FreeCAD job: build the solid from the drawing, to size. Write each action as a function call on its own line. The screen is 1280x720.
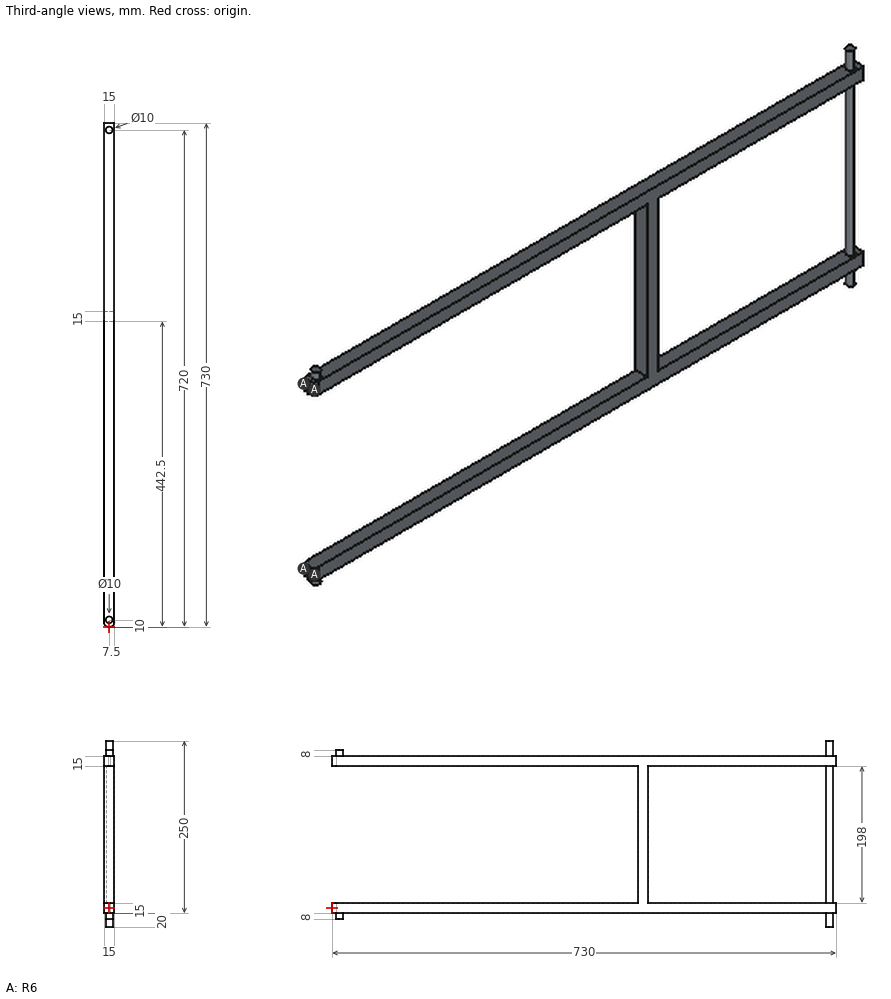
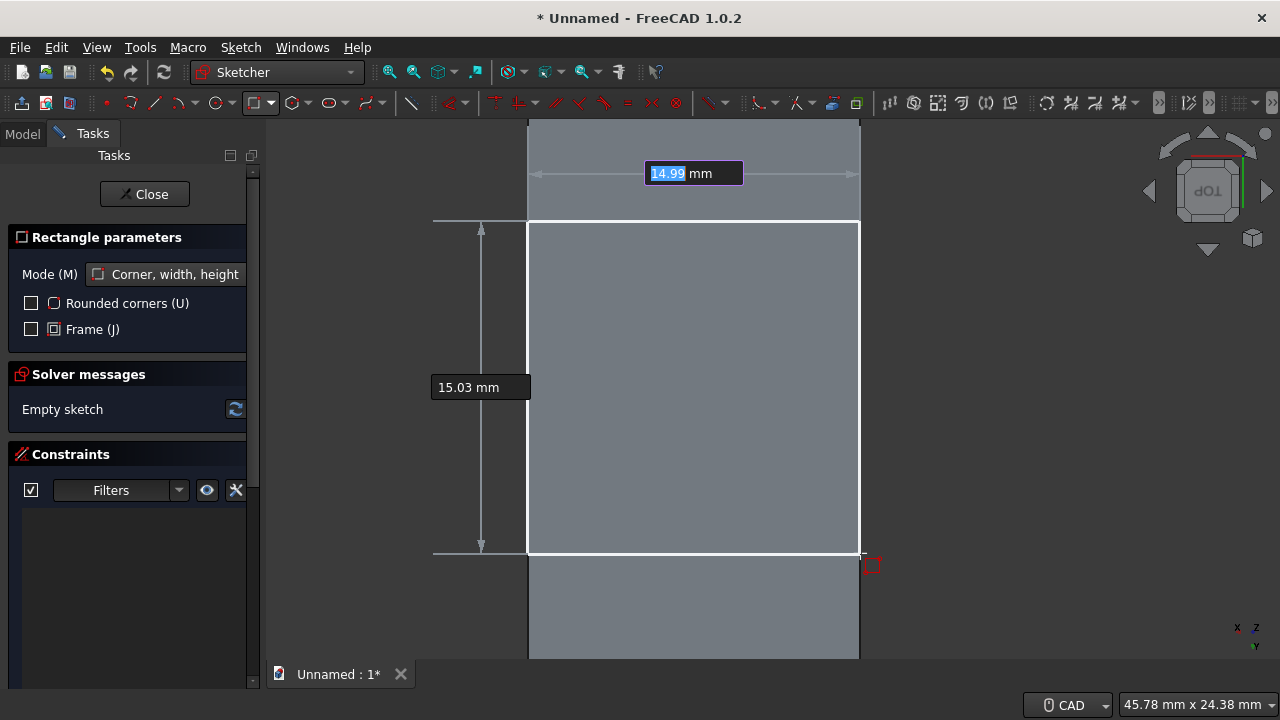
text(15)
key(Tab)
text(15)
key(Return)
key(Escape)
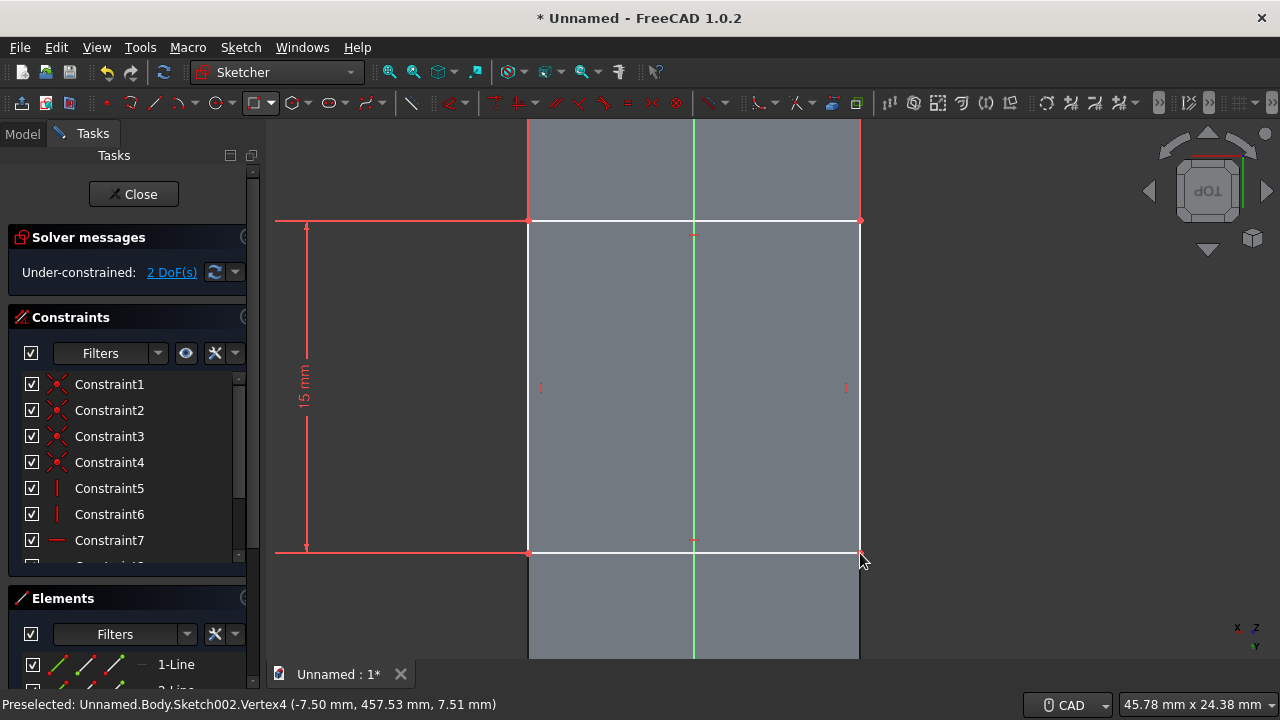
click(528, 221)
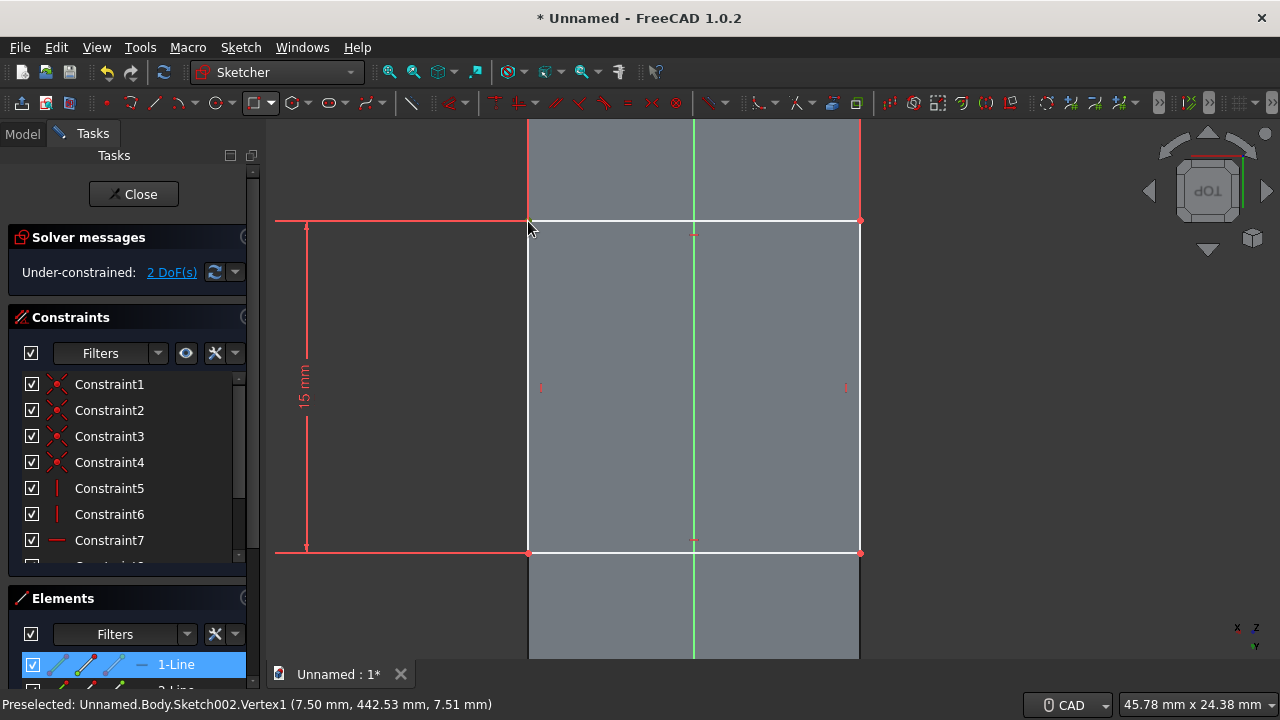
key(l)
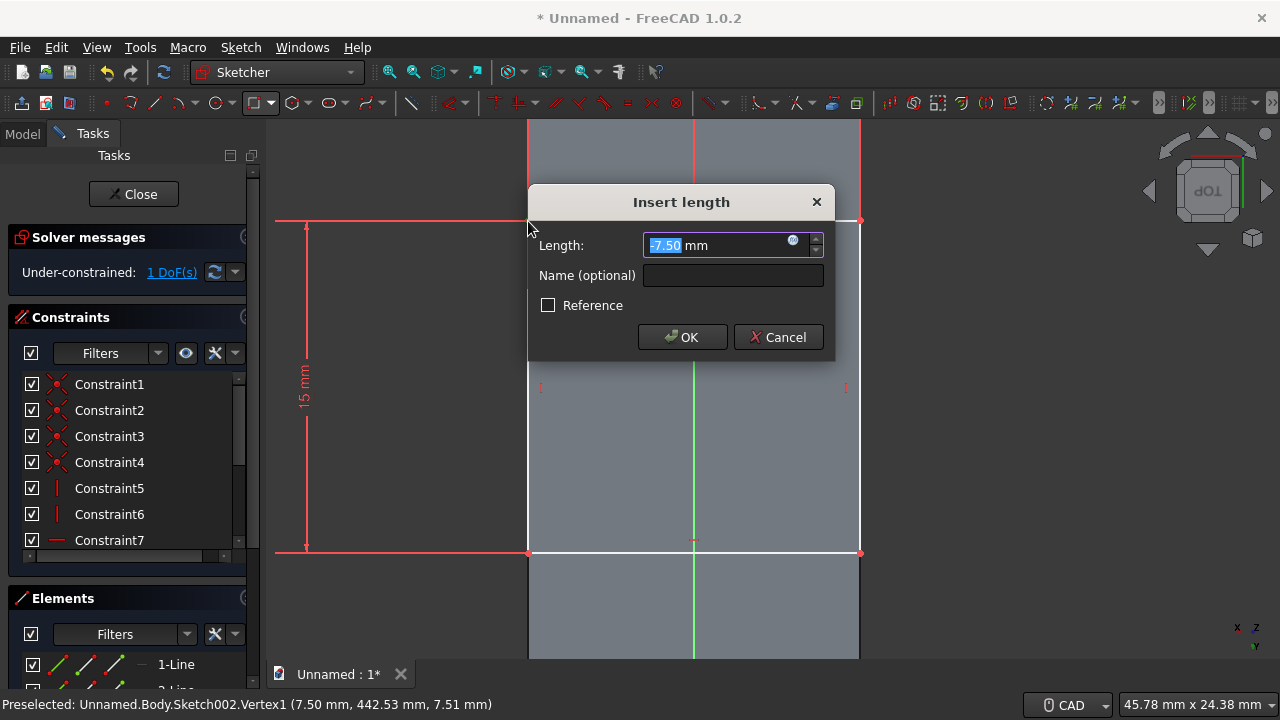
text(-7.5)
key(Return)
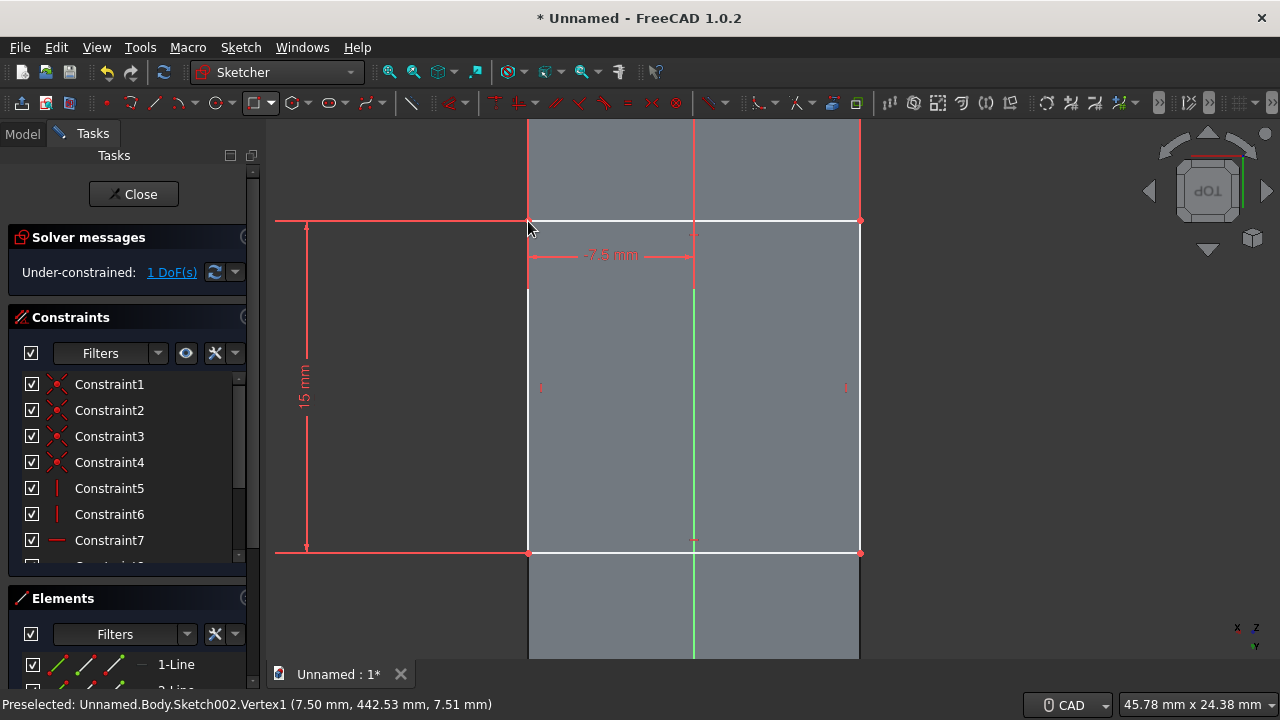
click(528, 221)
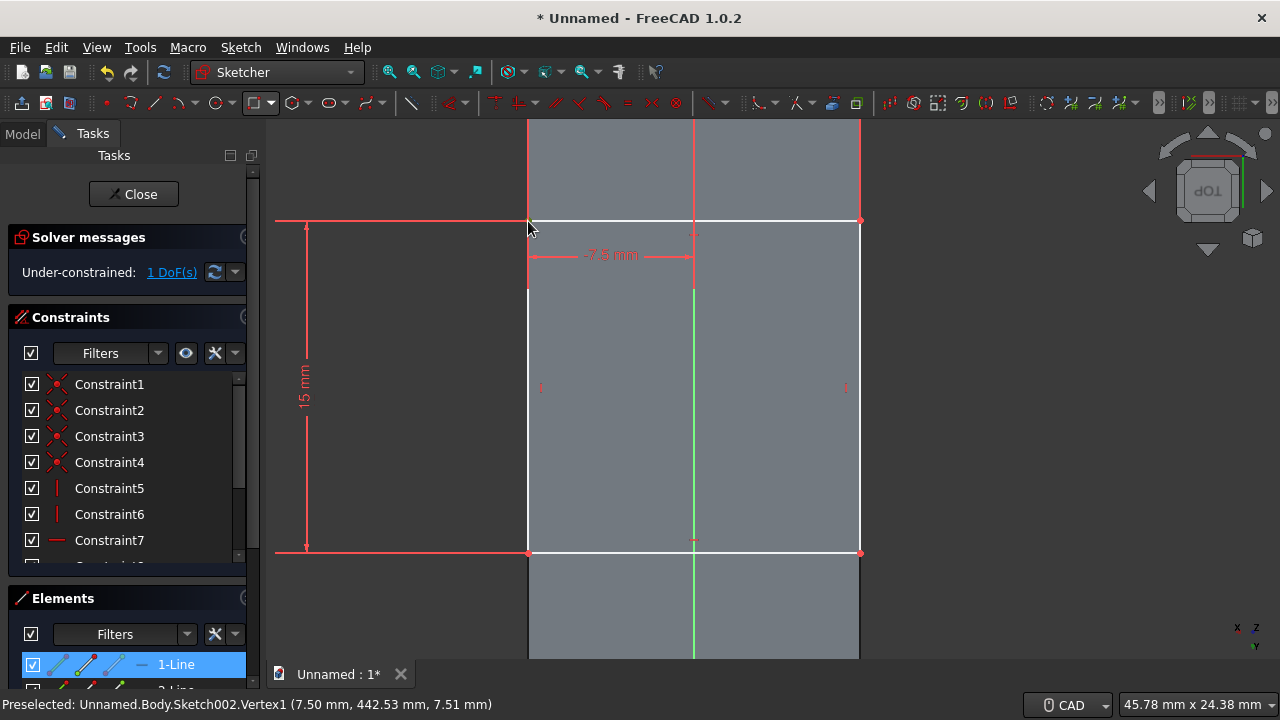
click(468, 104)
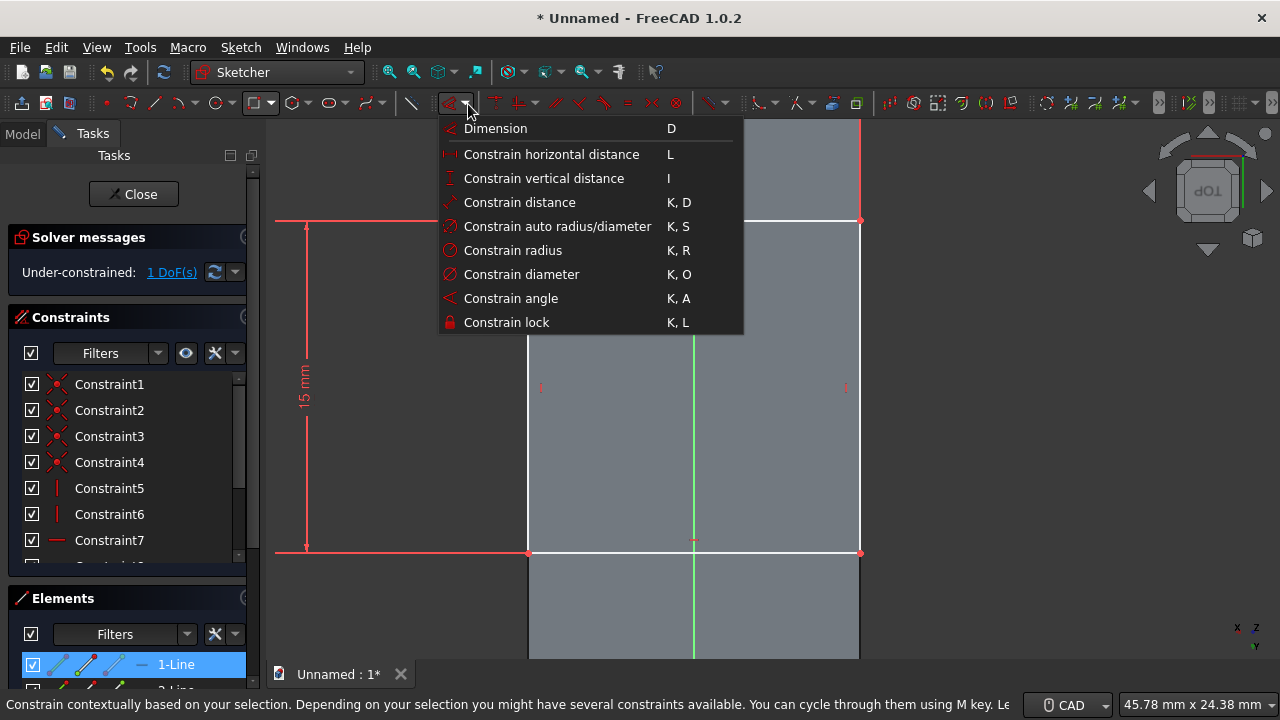
click(591, 178)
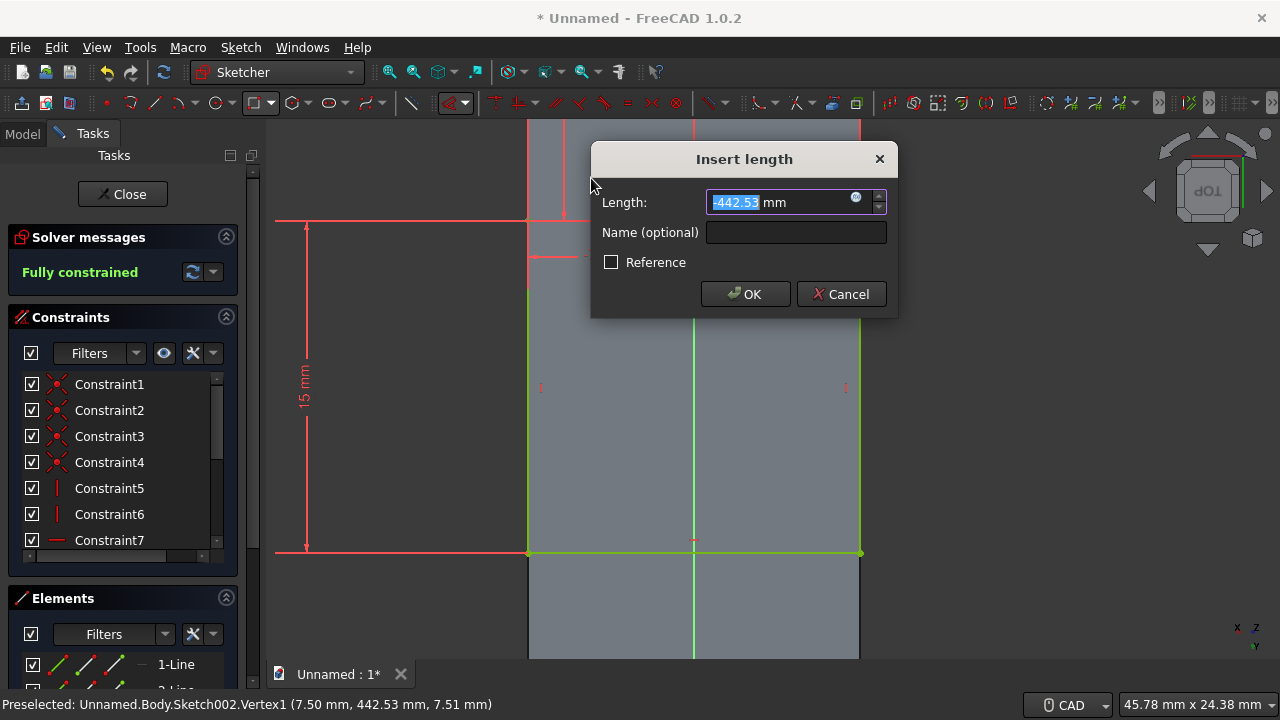
text(-442.5)
key(Return)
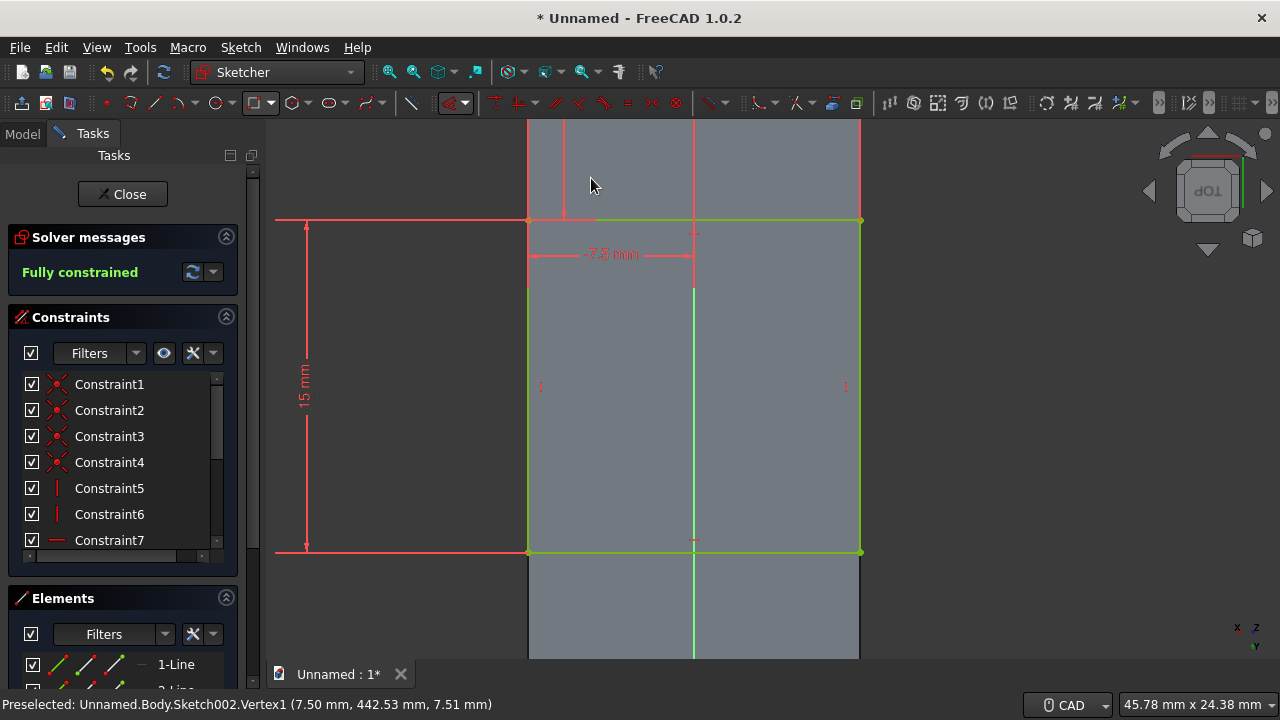
click(123, 194)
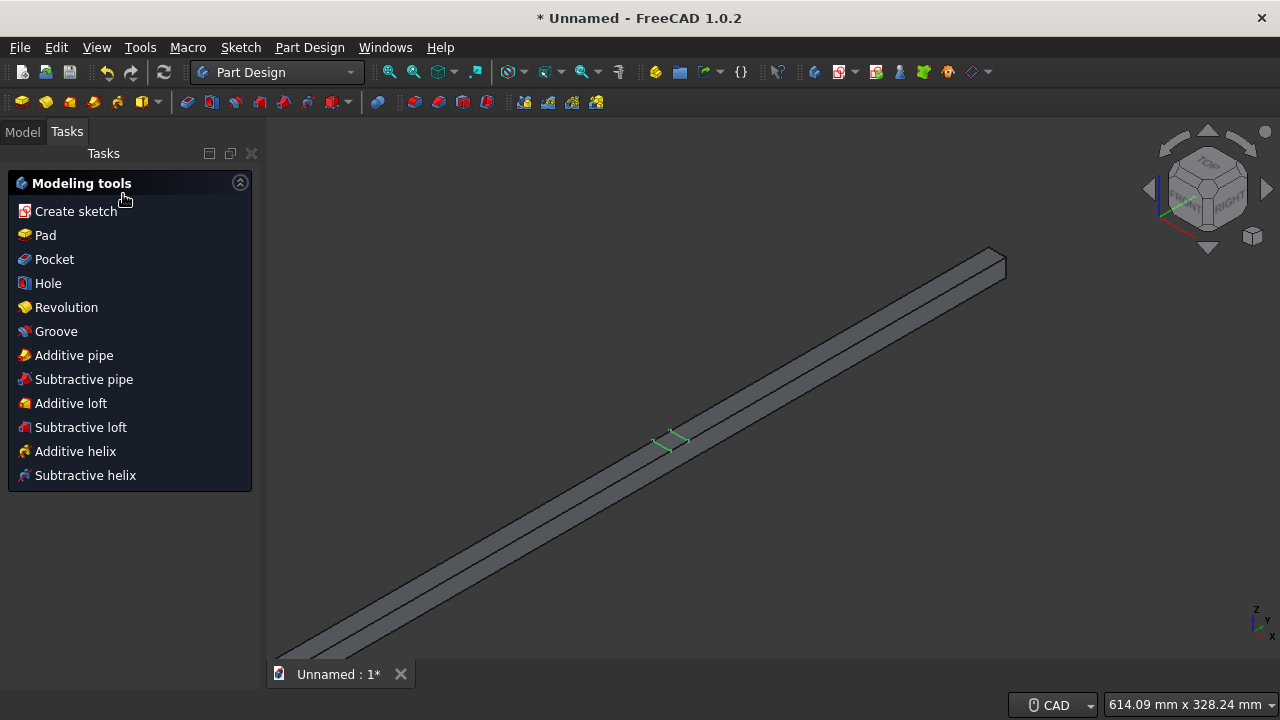
click(22, 102)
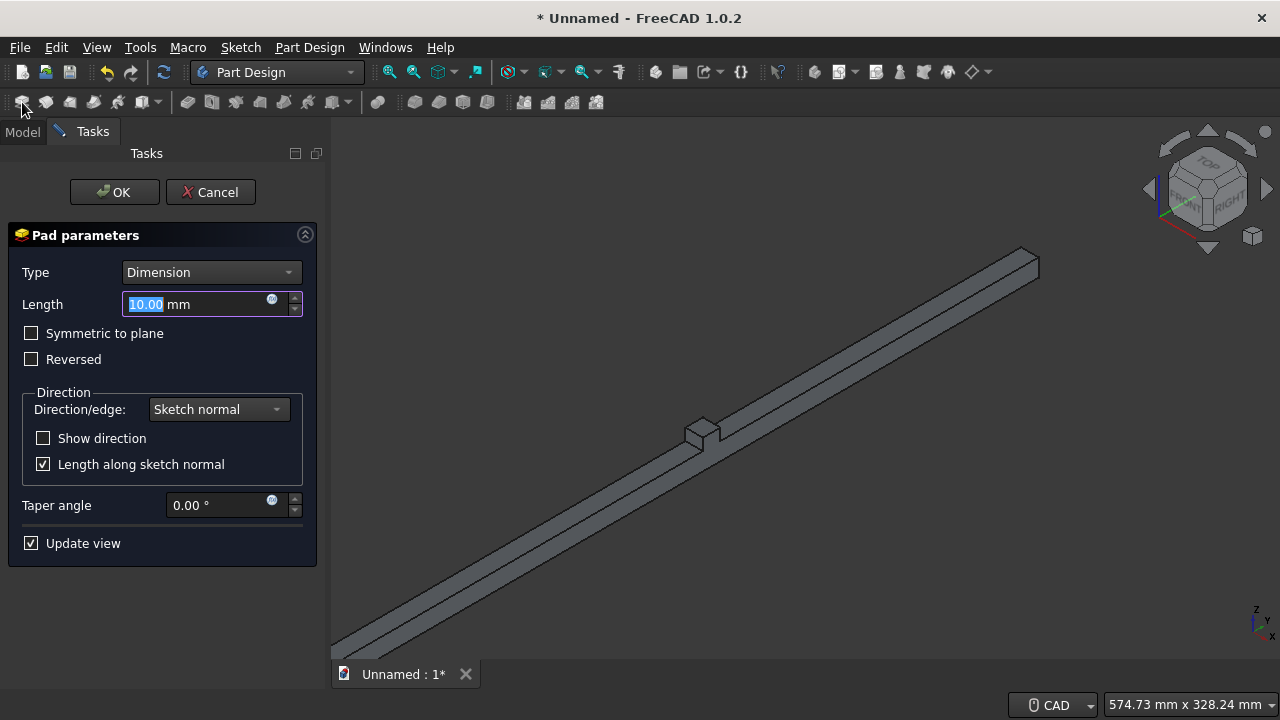
text(198)
key(Tab)